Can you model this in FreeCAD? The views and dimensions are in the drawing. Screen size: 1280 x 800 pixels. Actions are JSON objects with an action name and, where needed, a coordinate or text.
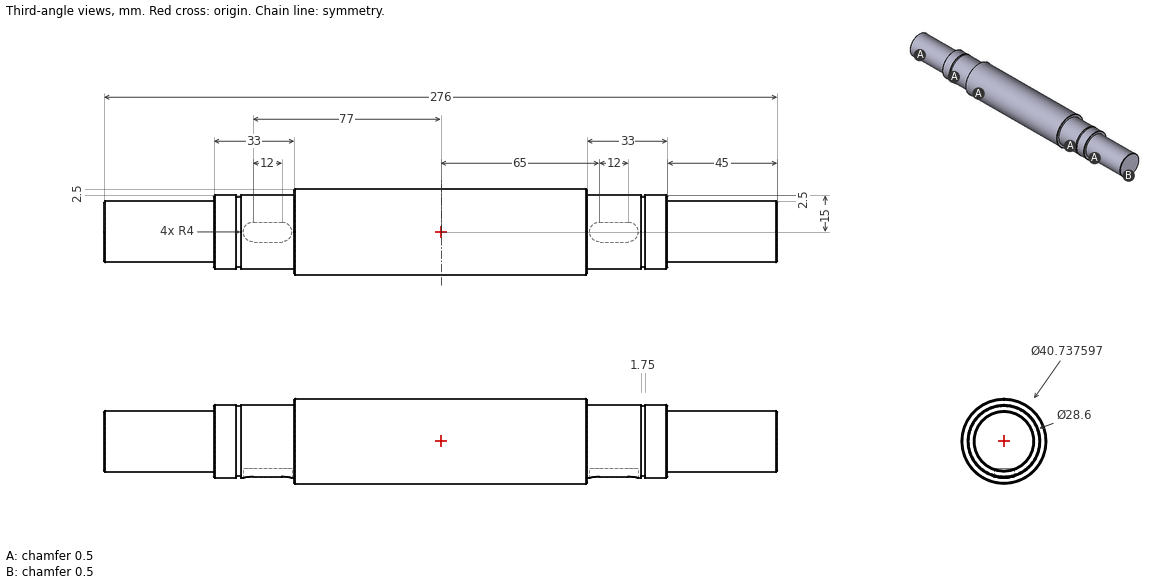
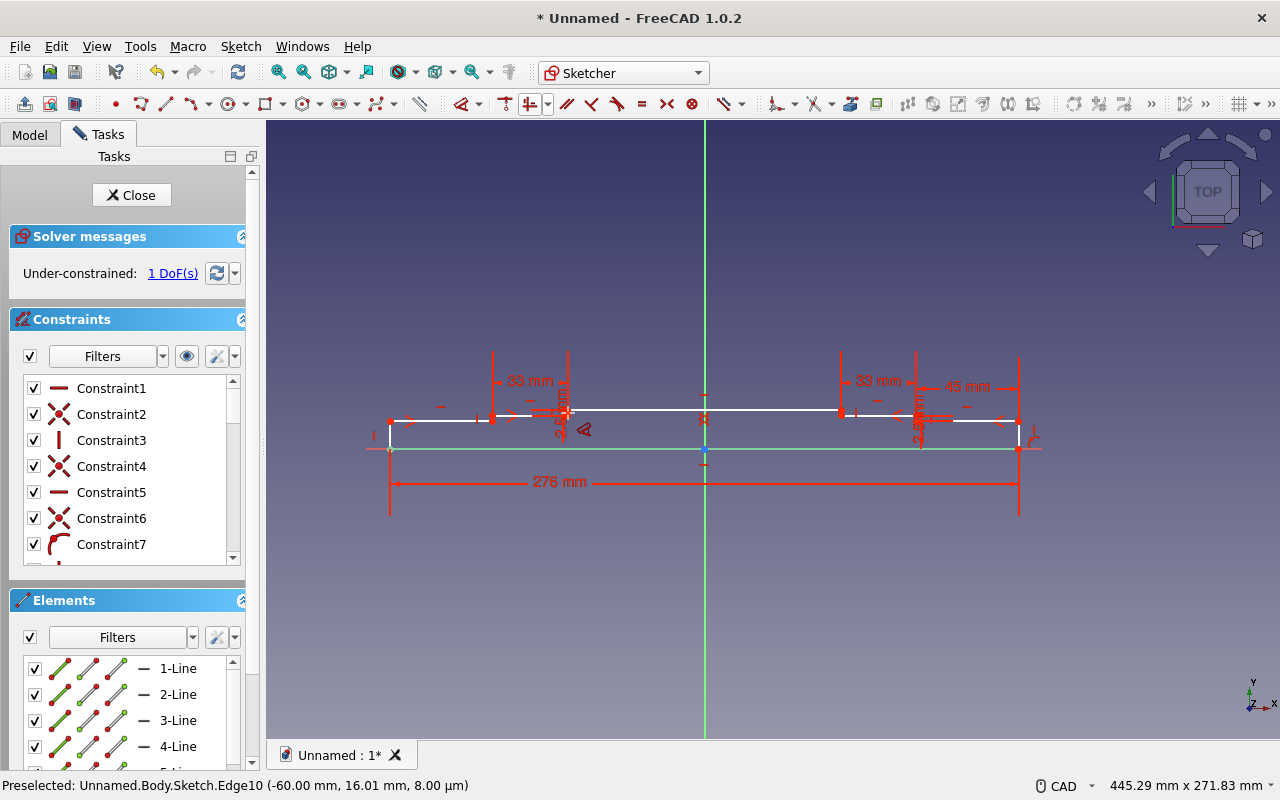
{"action": "scroll", "coordinate": [841, 416], "scroll_direction": "up", "scroll_amount": 4}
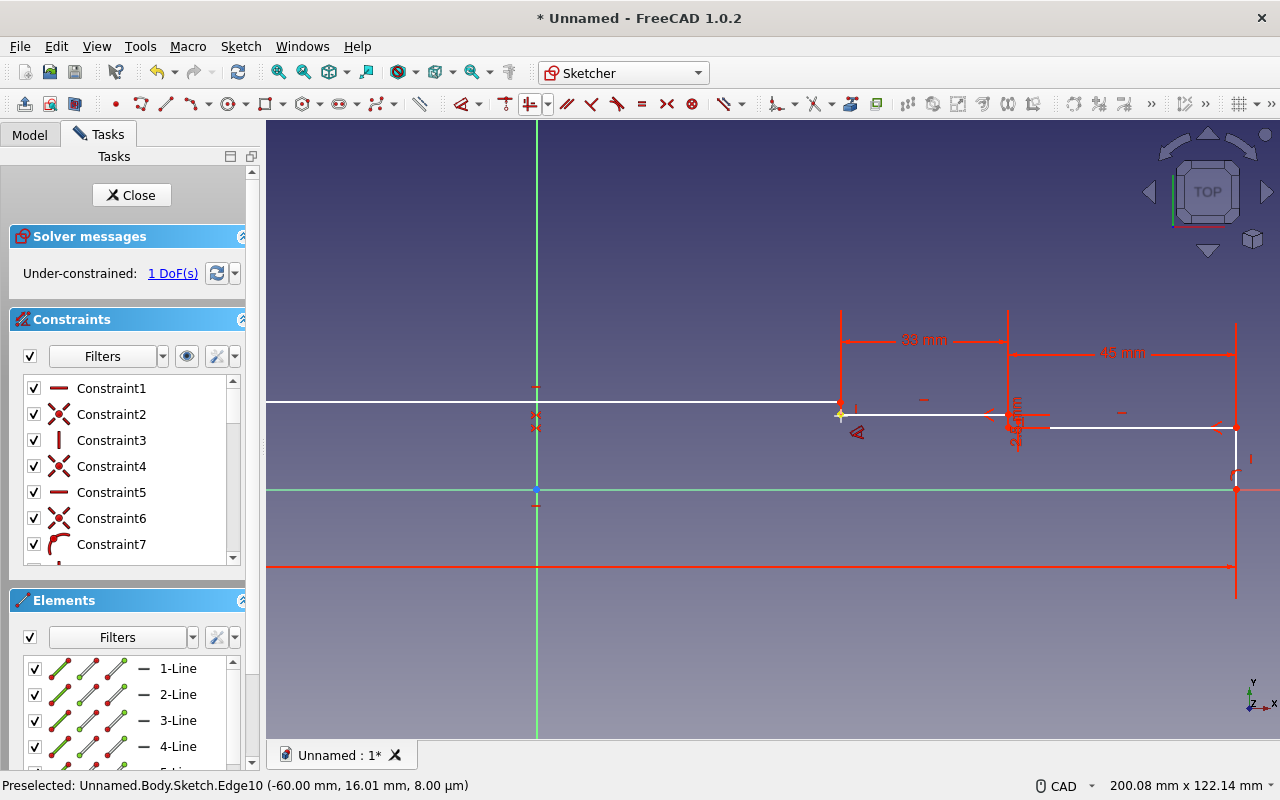
{"action": "left_click", "coordinate": [841, 415]}
{"action": "left_click", "coordinate": [875, 452]}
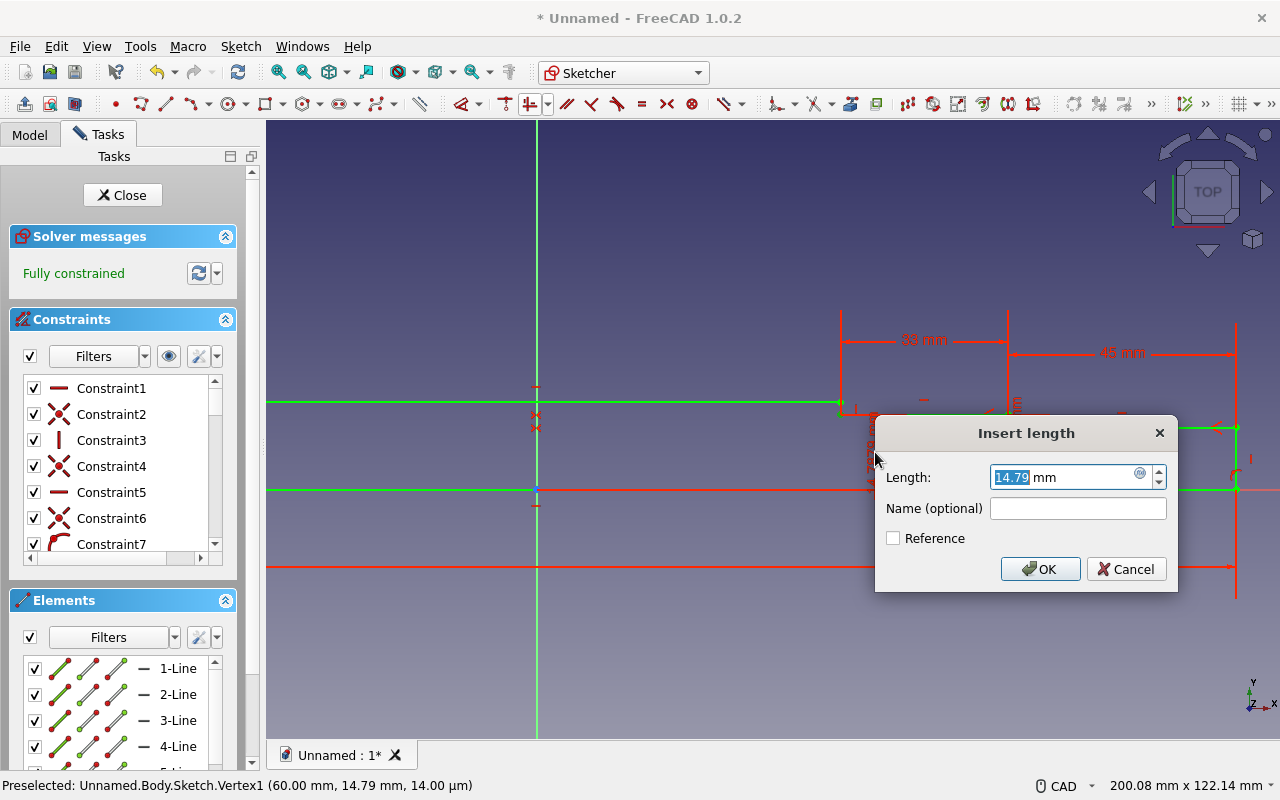
{"action": "type", "text": "15"}
{"action": "key", "text": "Return"}
{"action": "key", "text": "Escape"}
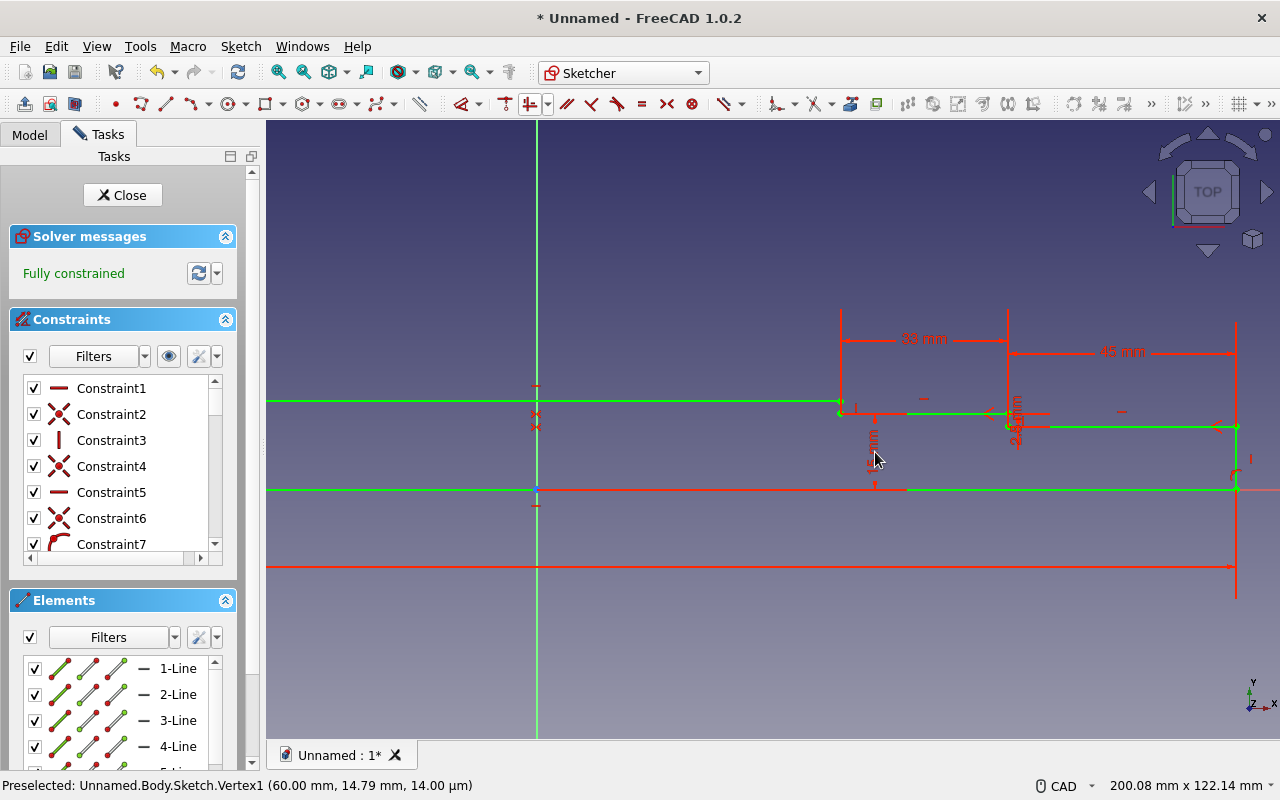
{"action": "left_click", "coordinate": [123, 195]}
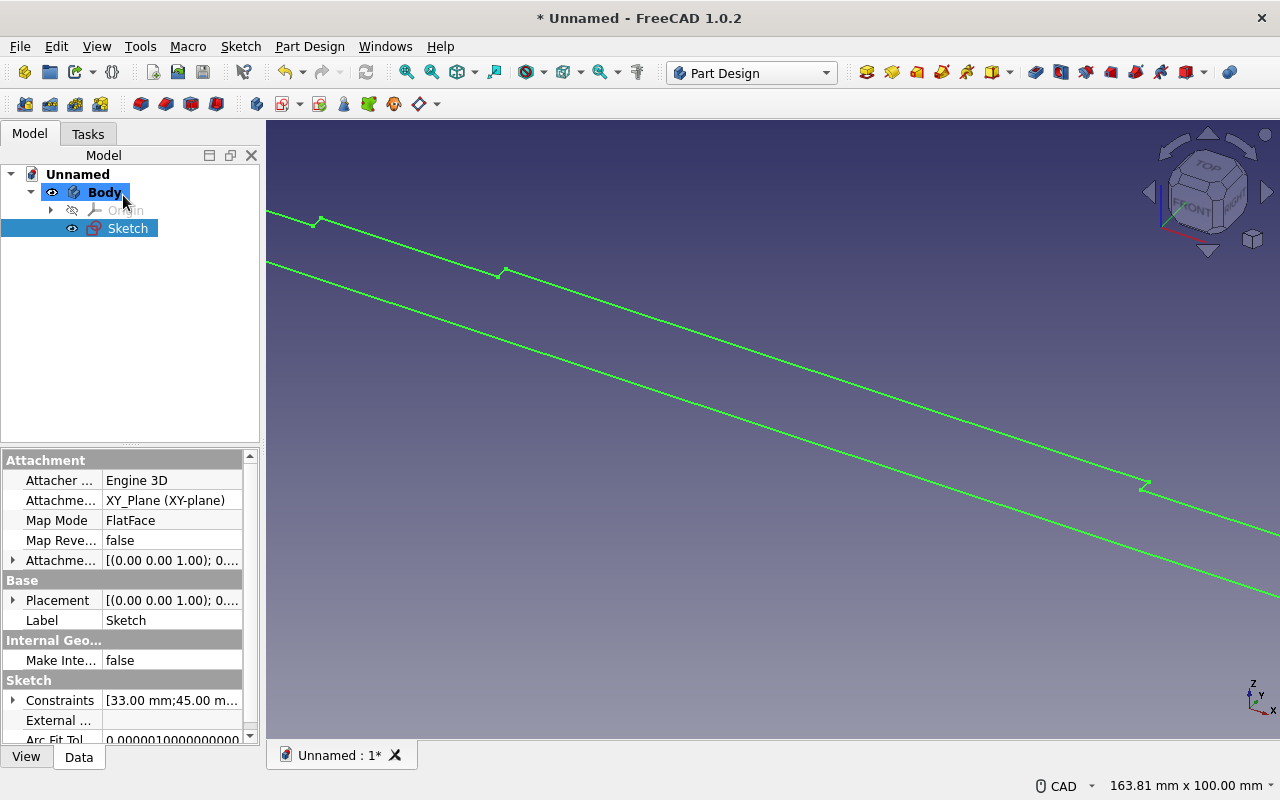
{"action": "left_click", "coordinate": [892, 72]}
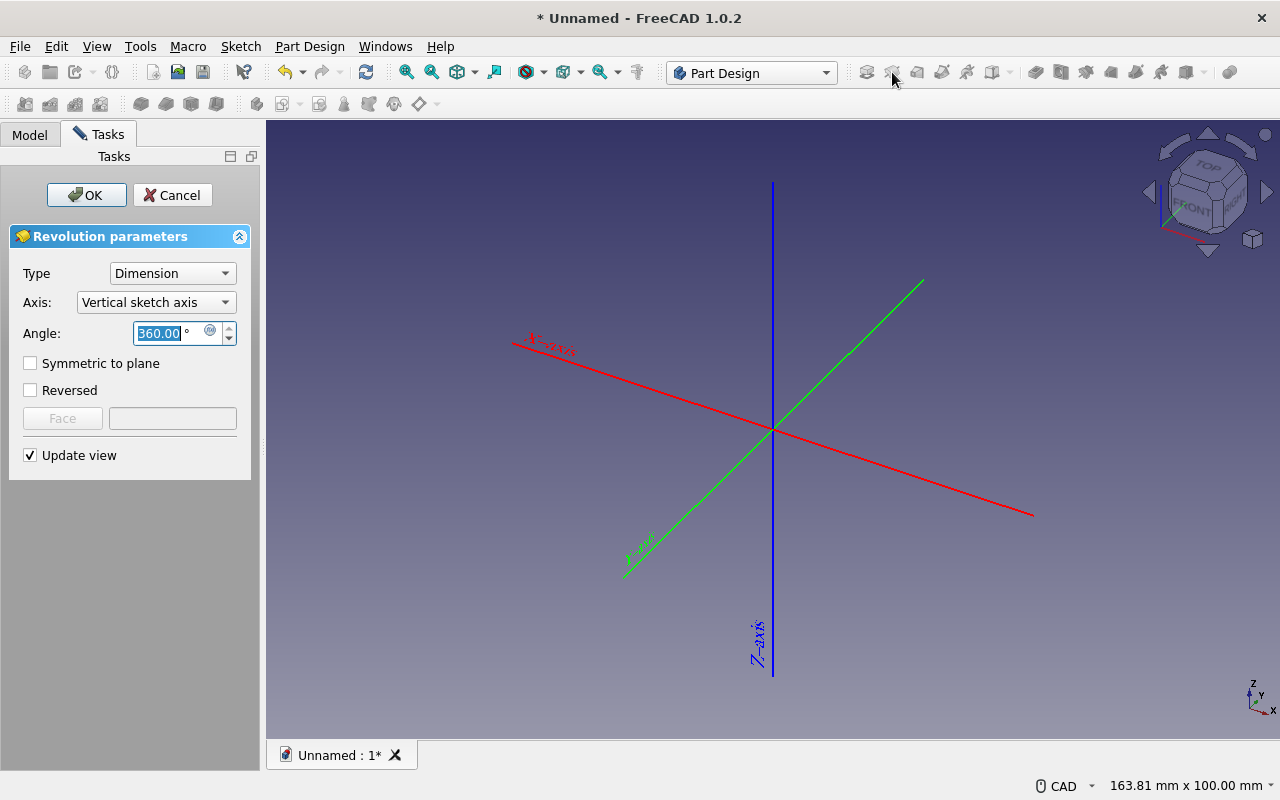
{"action": "left_click", "coordinate": [157, 302]}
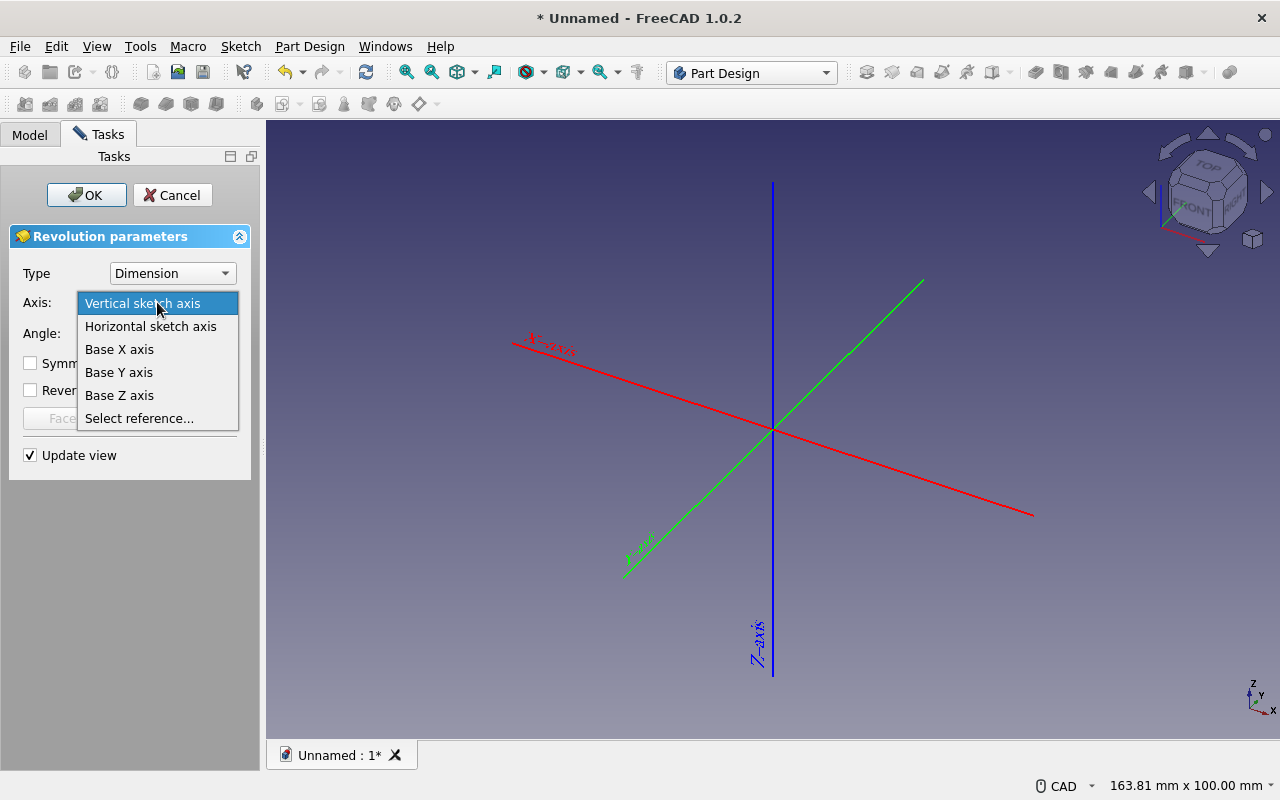
{"action": "left_click", "coordinate": [156, 326]}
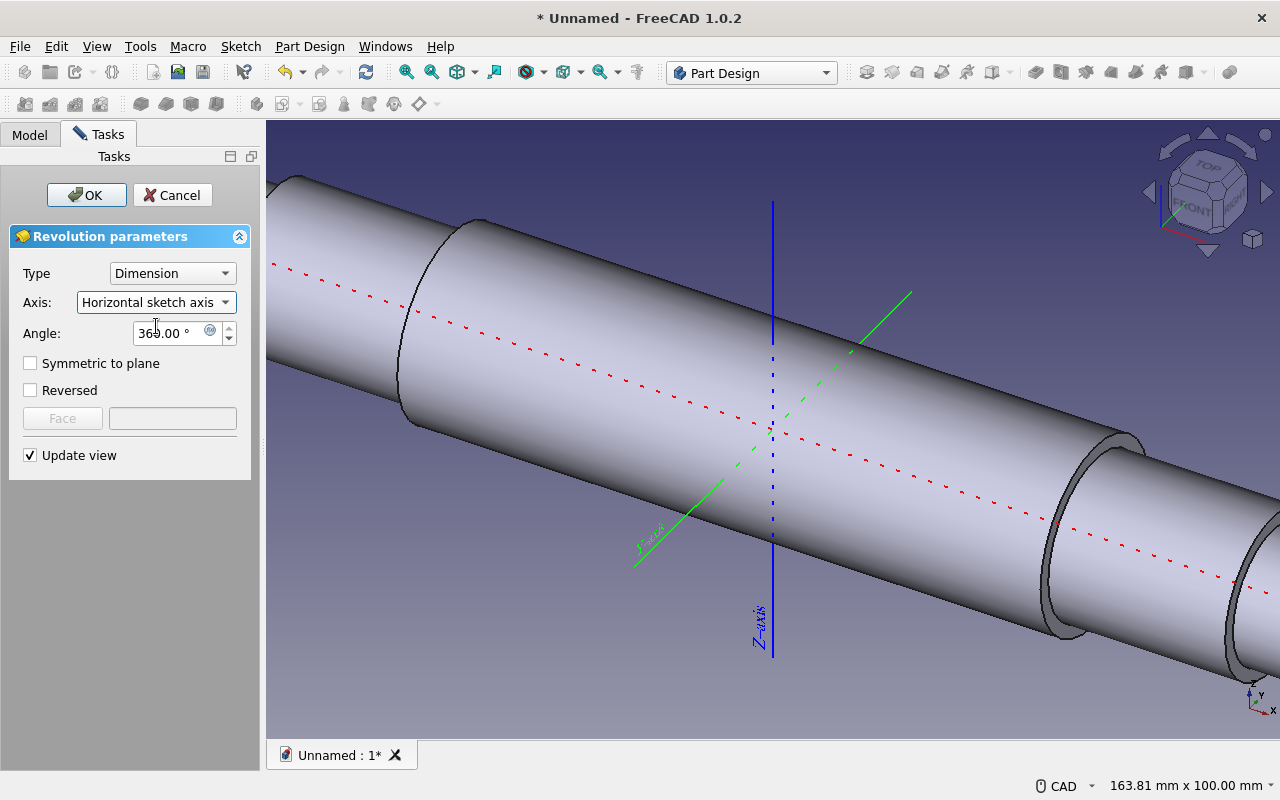
{"action": "left_click", "coordinate": [87, 195]}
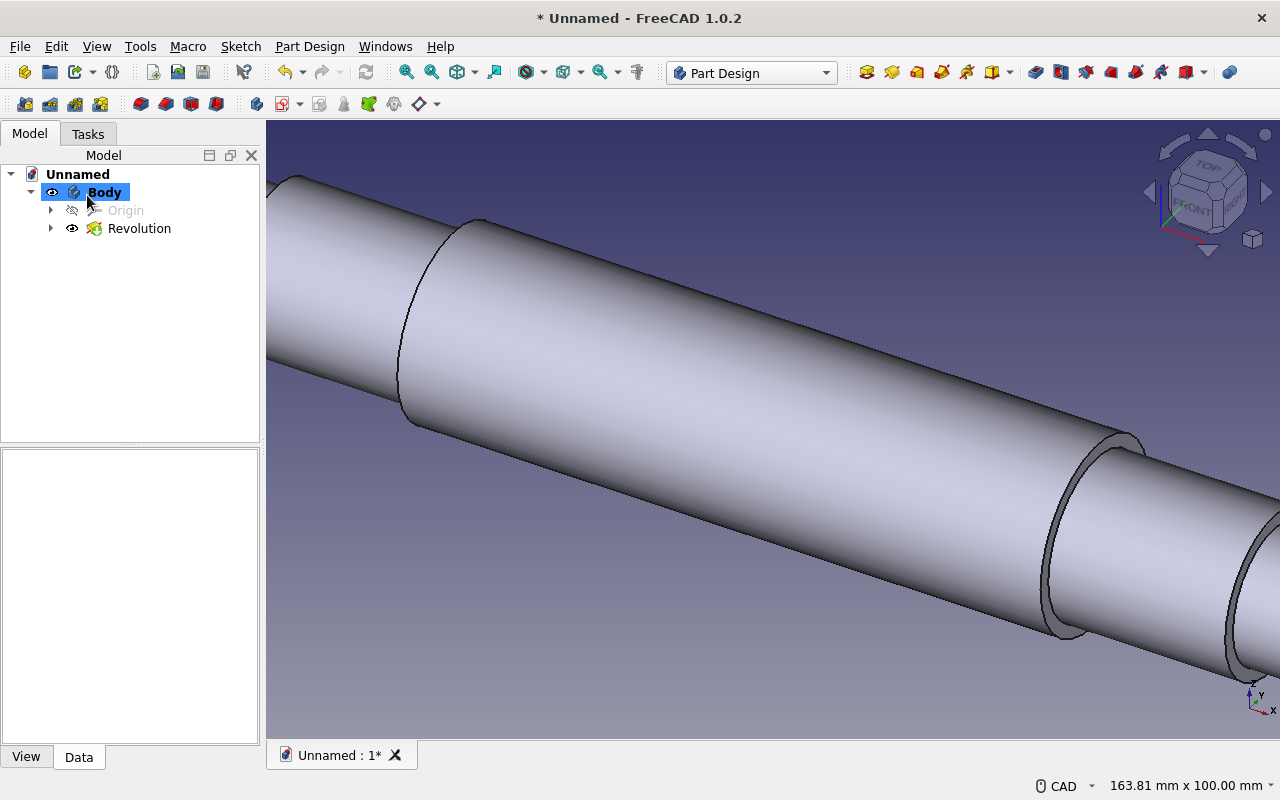
{"action": "left_click", "coordinate": [407, 72]}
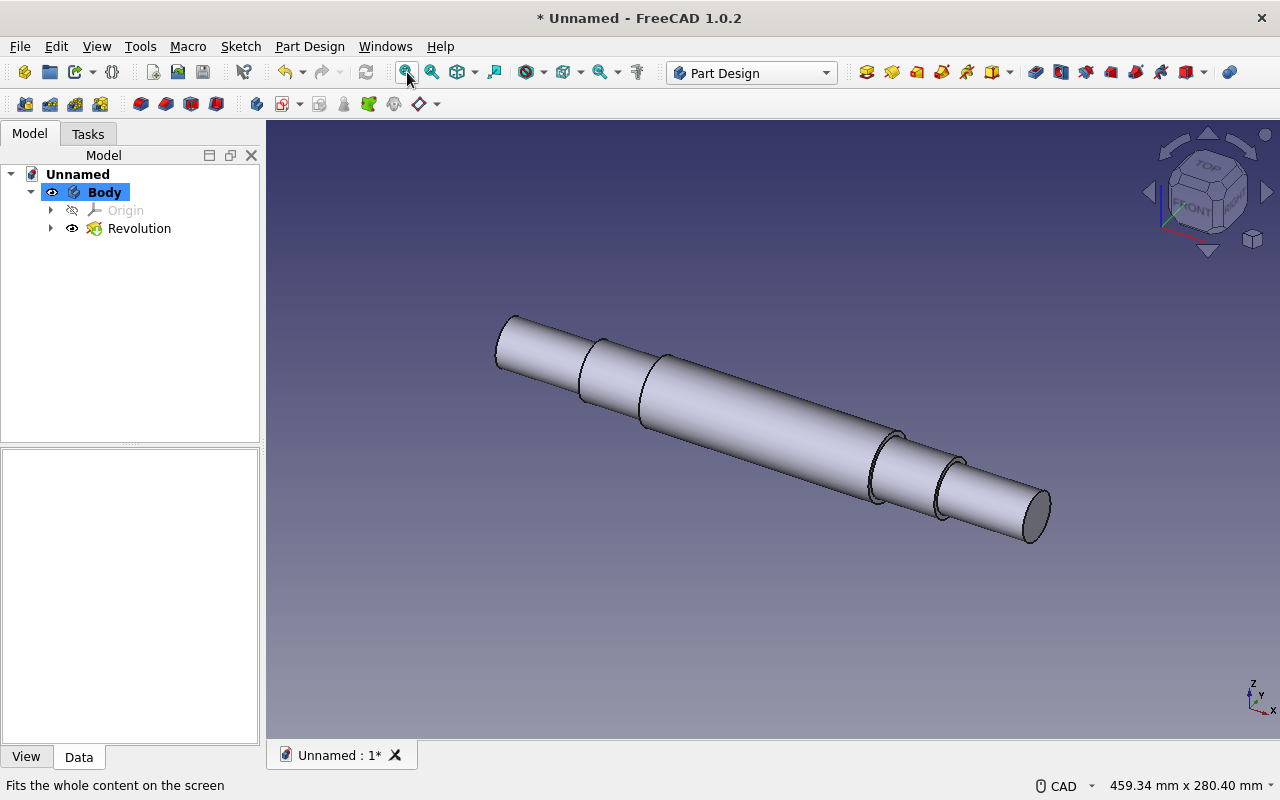
{"action": "left_click", "coordinate": [498, 366]}